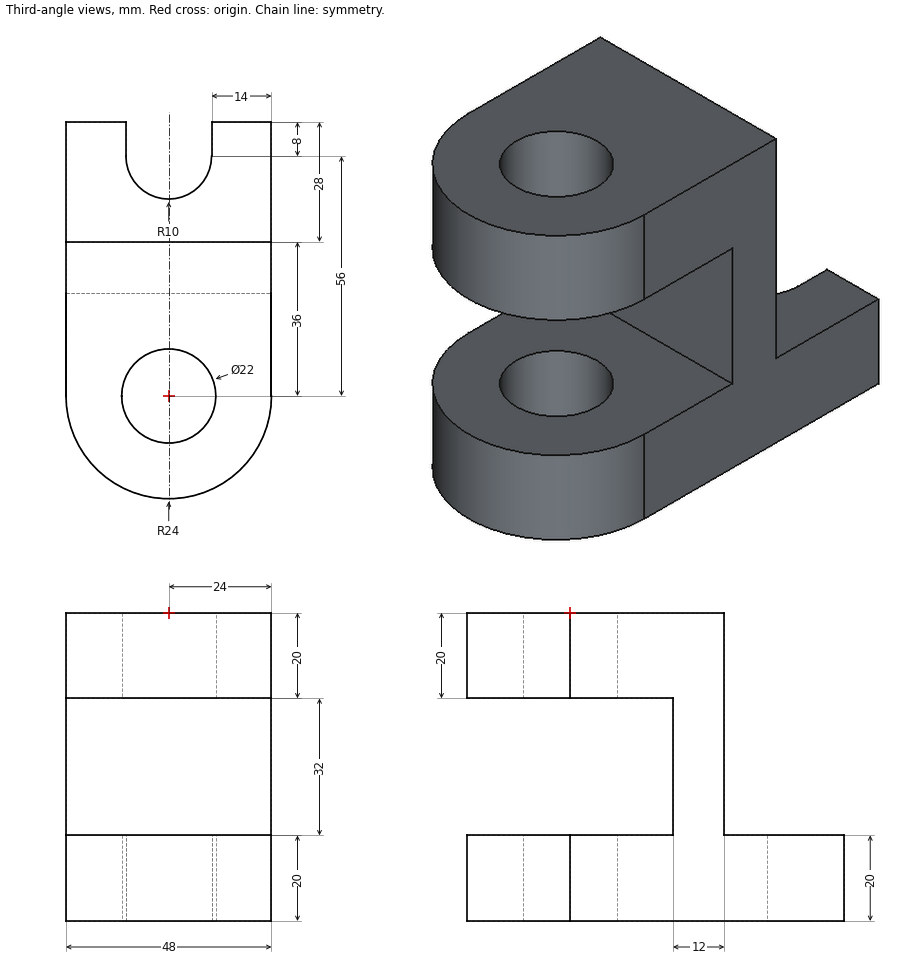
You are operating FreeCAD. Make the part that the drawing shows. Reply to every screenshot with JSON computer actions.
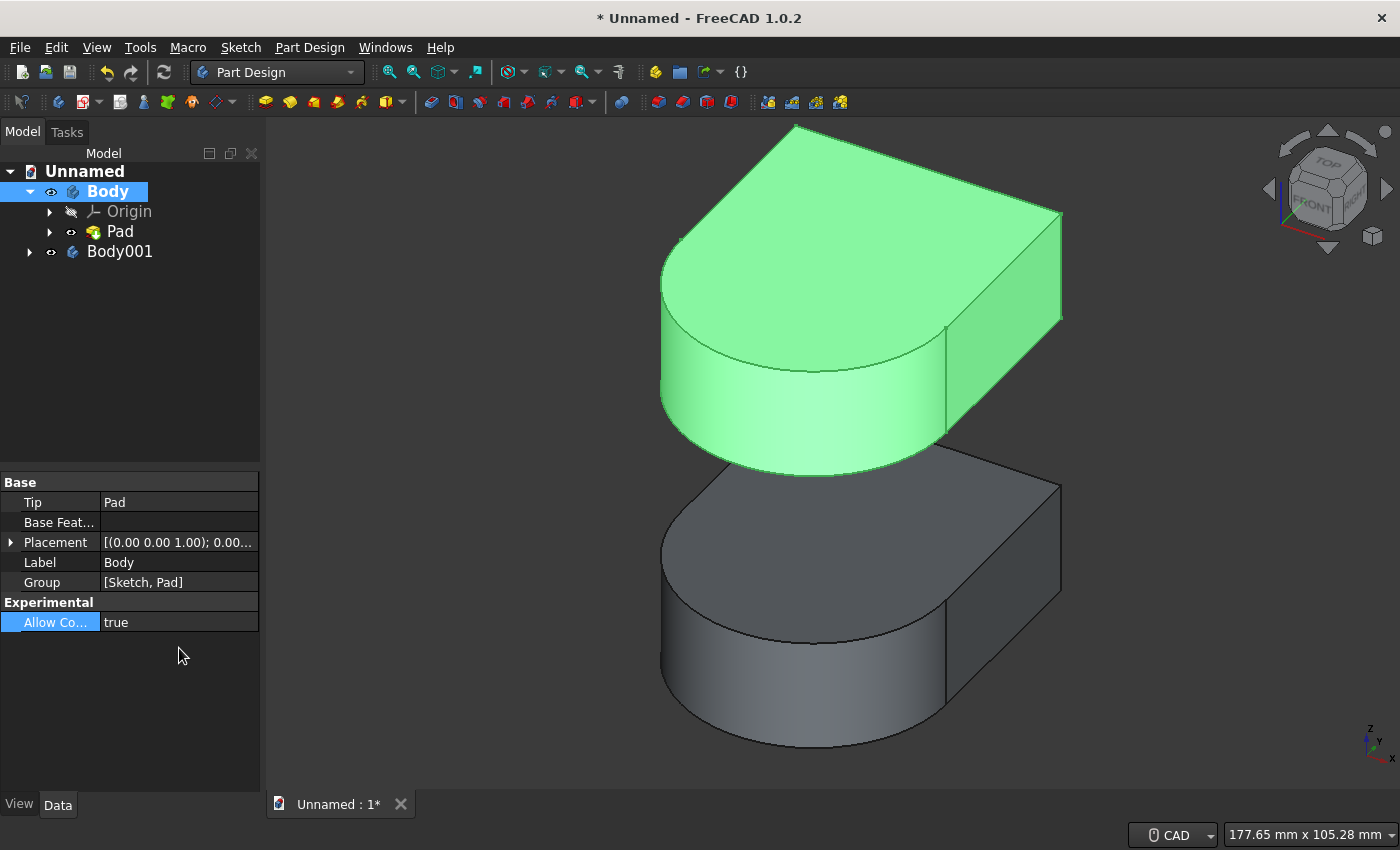
{"action": "left_click", "coordinate": [96, 252]}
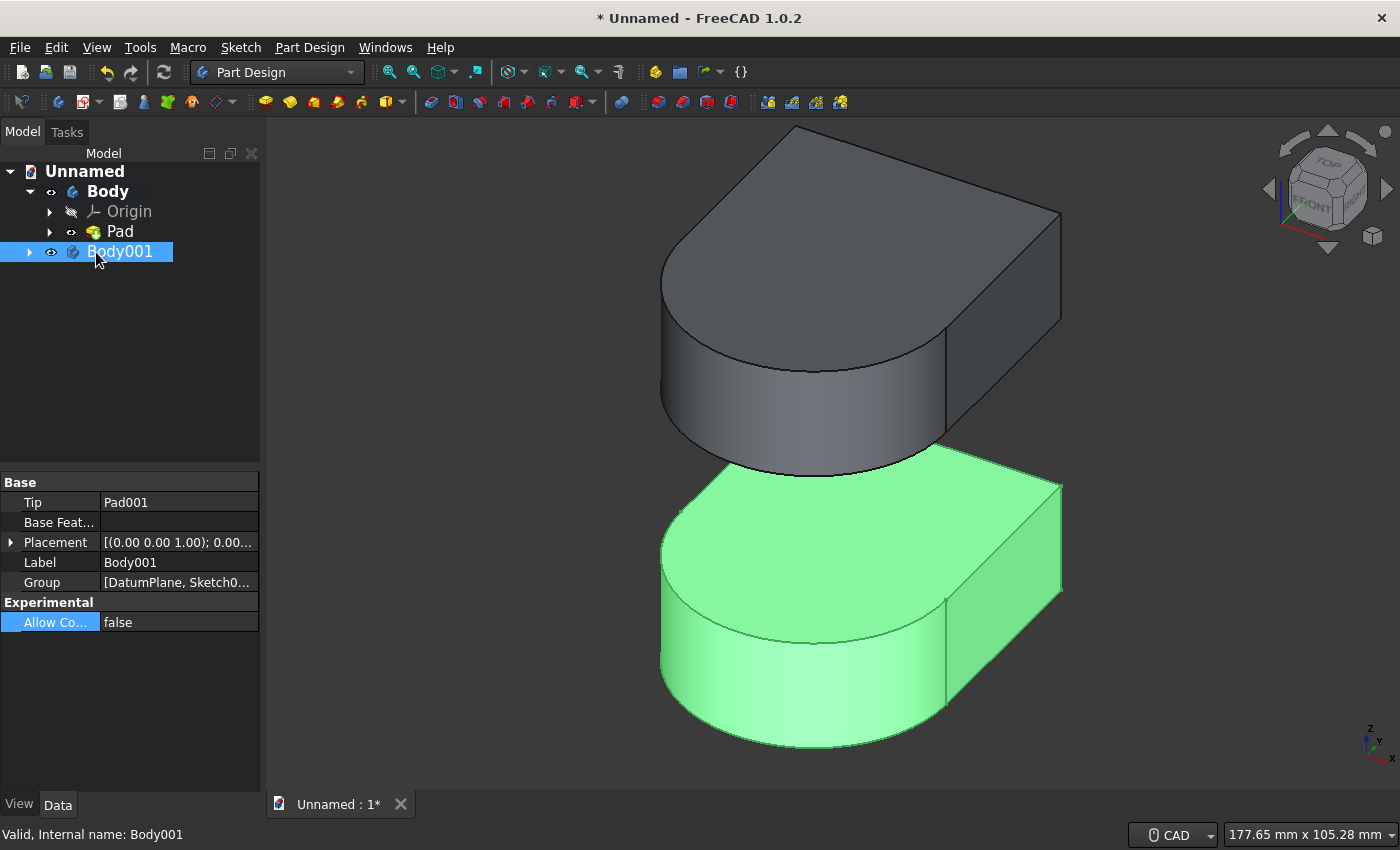
{"action": "left_click", "coordinate": [622, 102]}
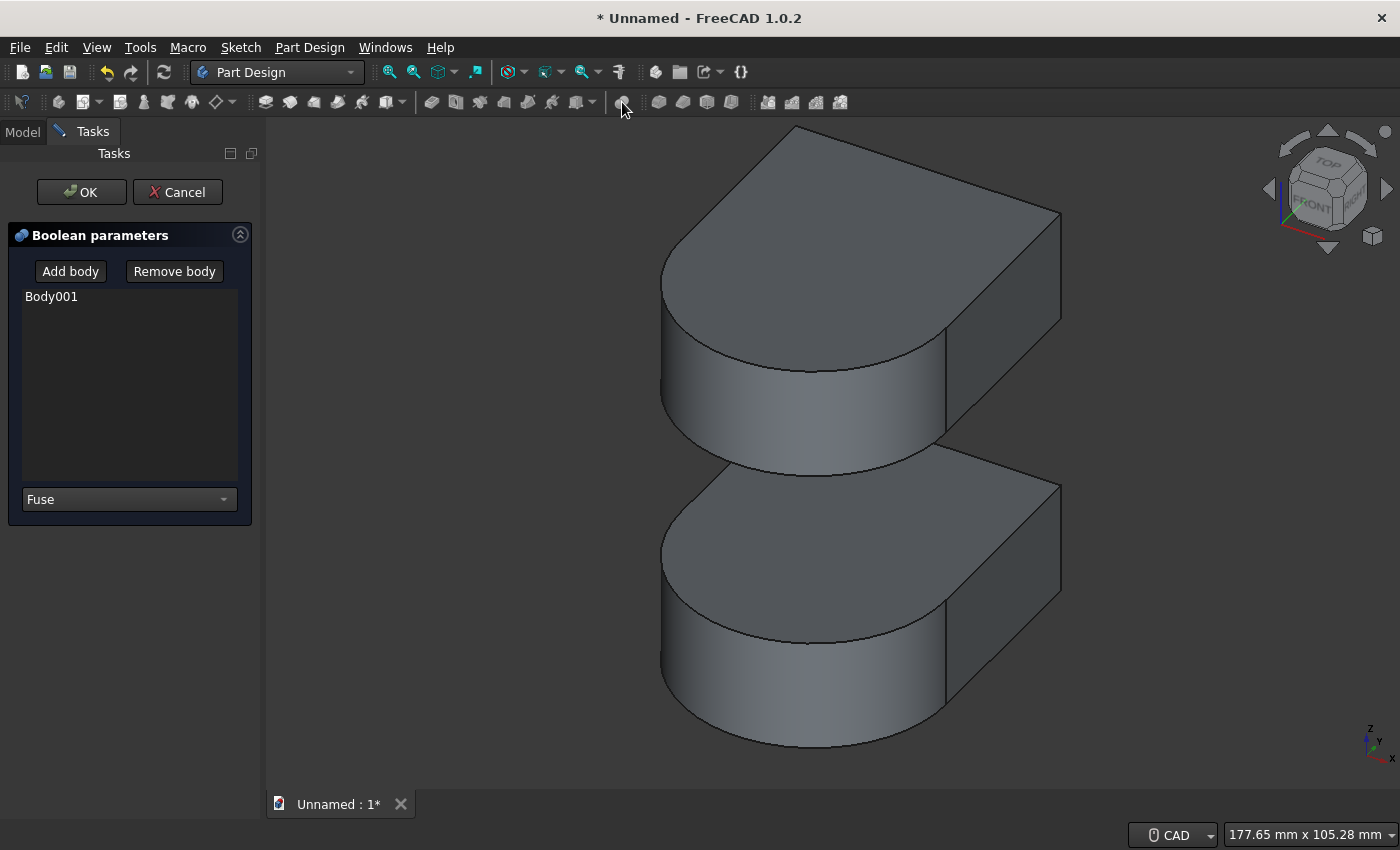
{"action": "left_click", "coordinate": [82, 192]}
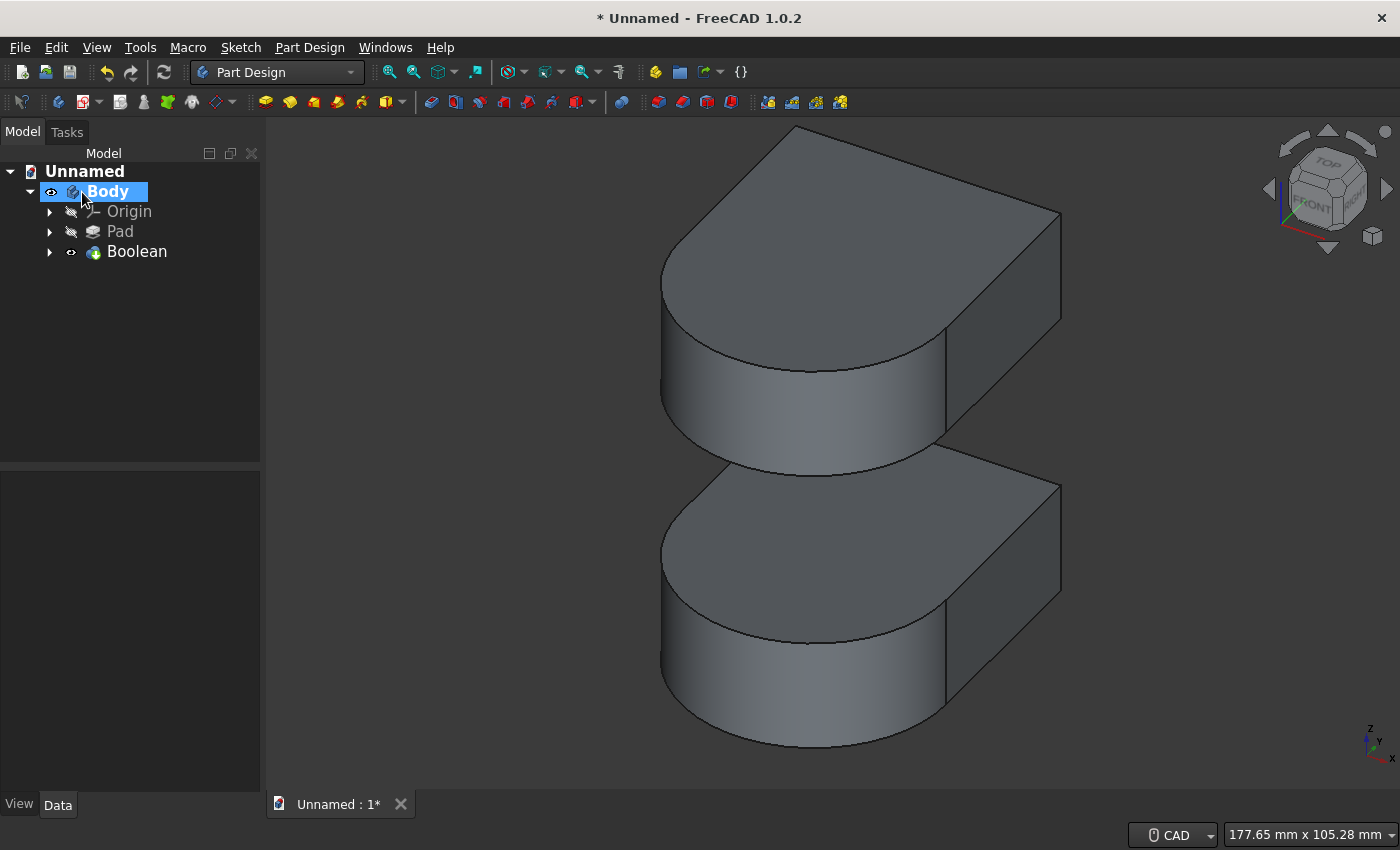
{"action": "key", "text": "4"}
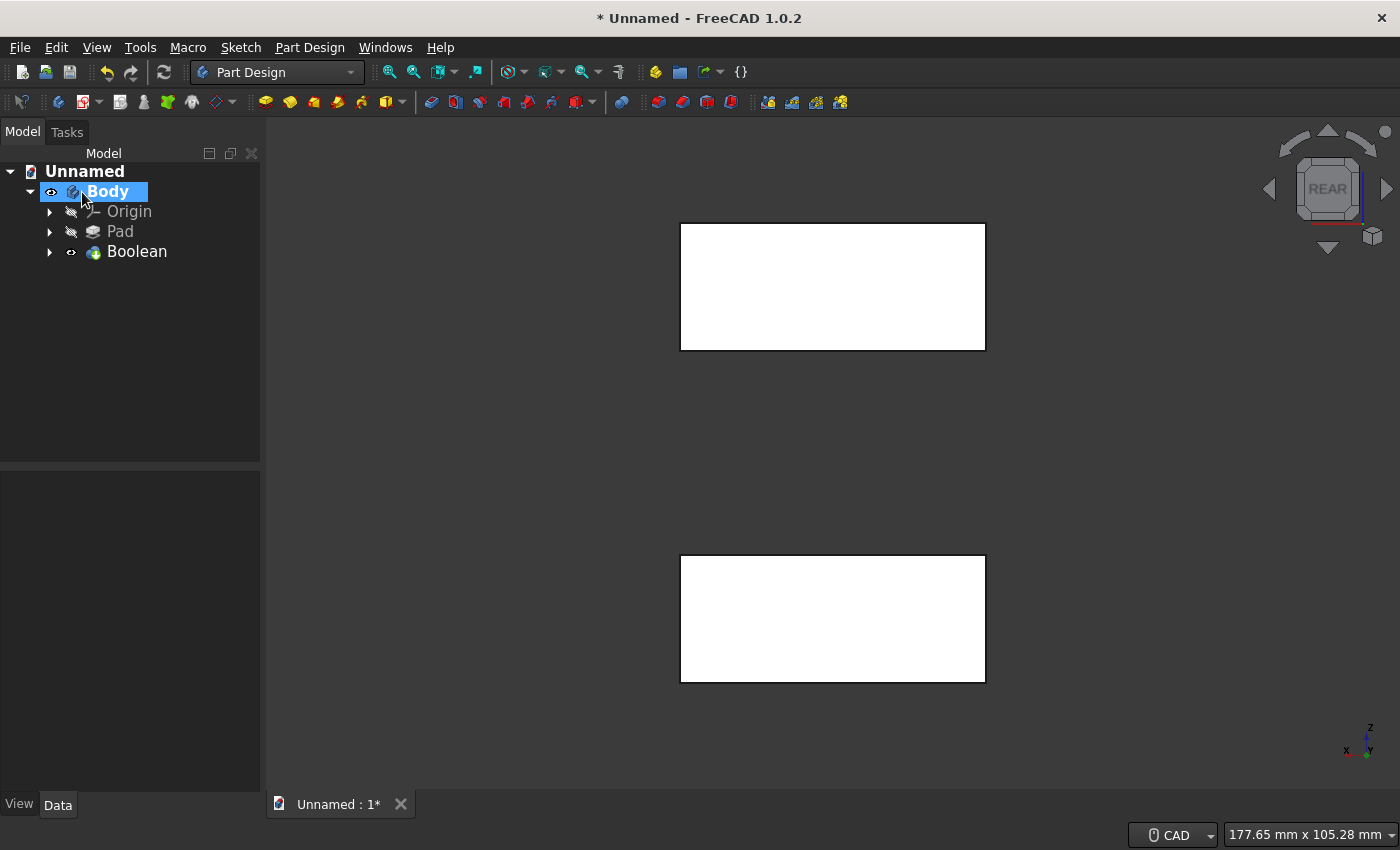
{"action": "left_click", "coordinate": [745, 618]}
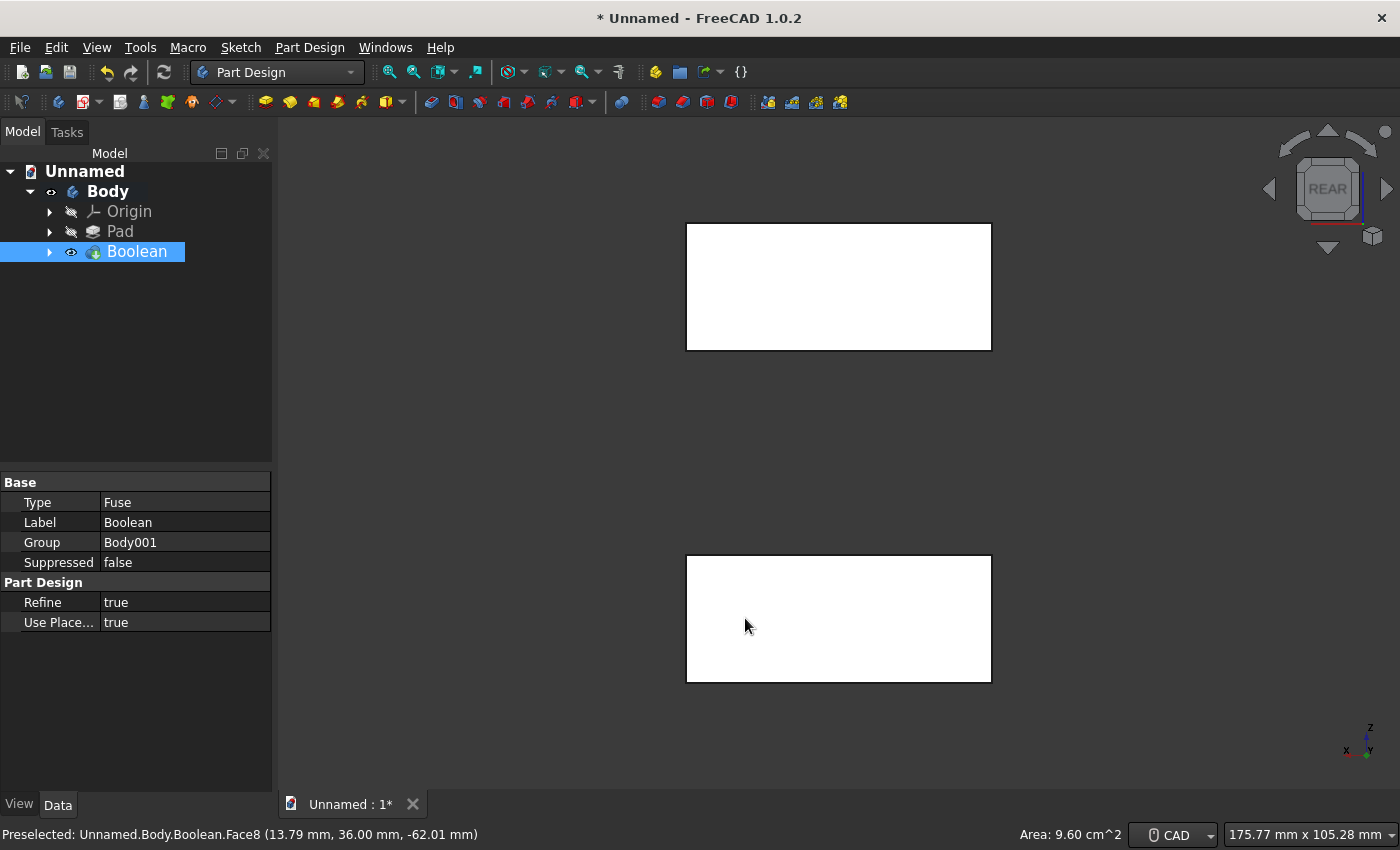
{"action": "left_click", "coordinate": [84, 102]}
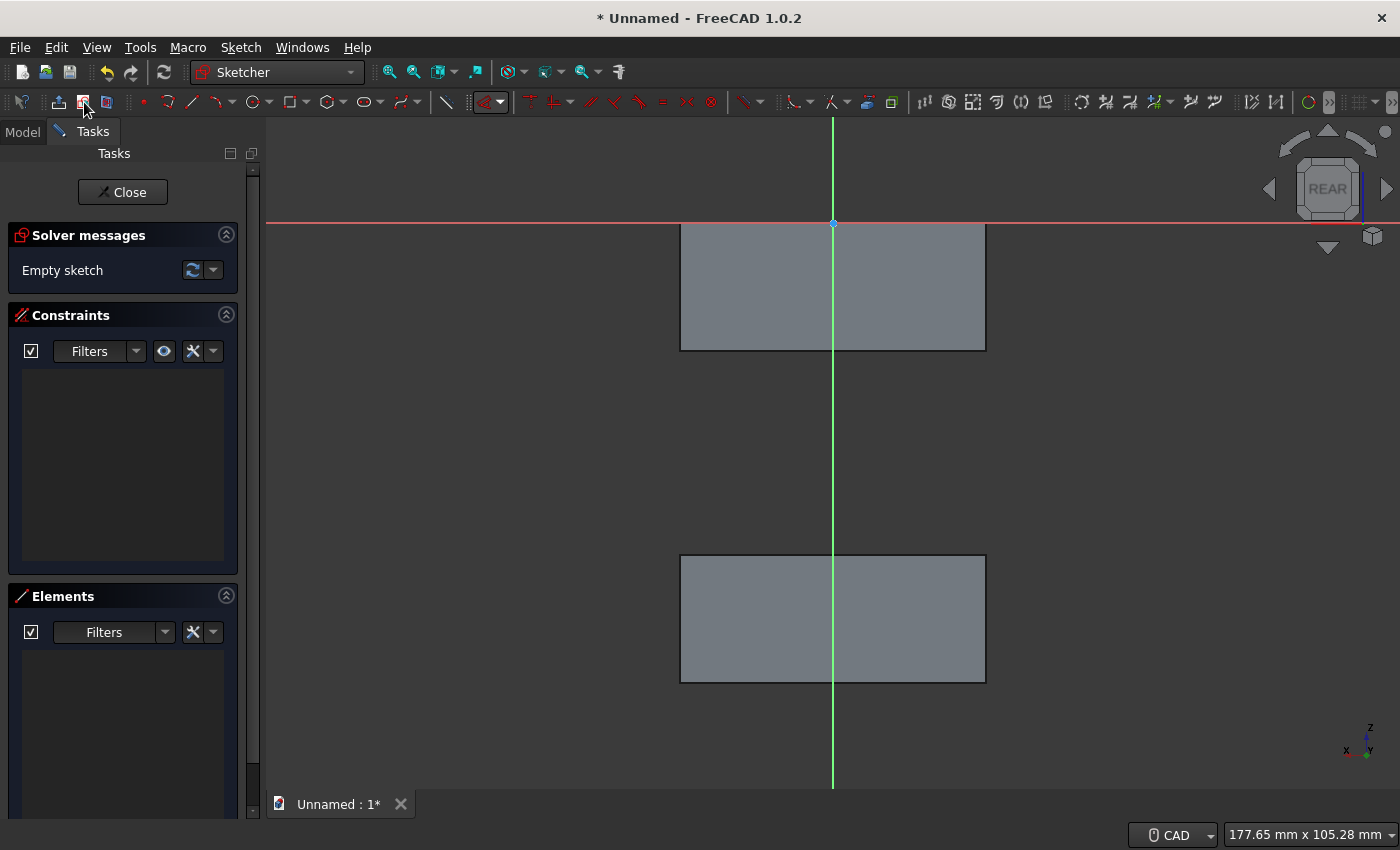
{"action": "left_click", "coordinate": [290, 102]}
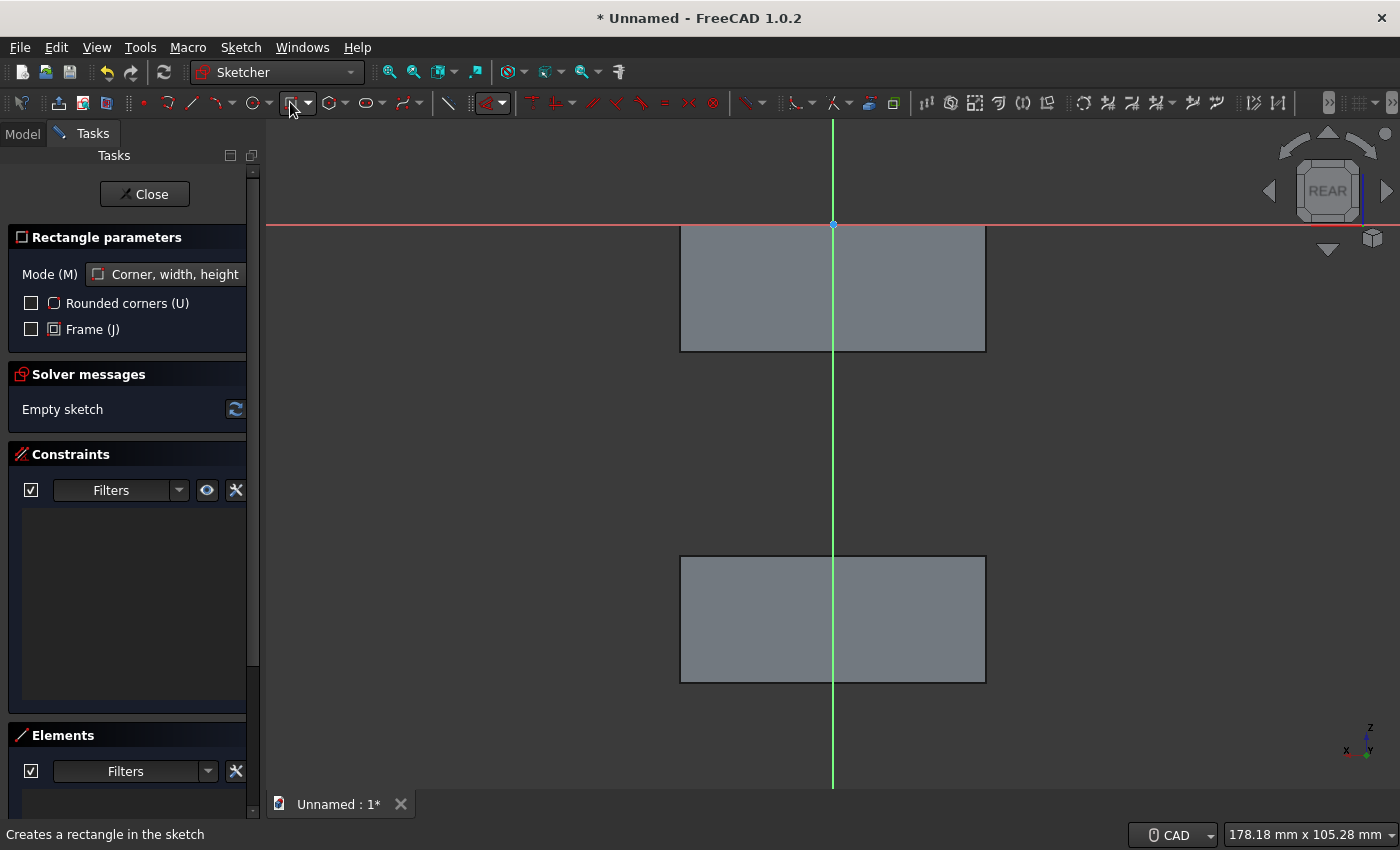
{"action": "left_click", "coordinate": [680, 352]}
{"action": "left_click", "coordinate": [986, 556]}
{"action": "key", "text": "Escape"}